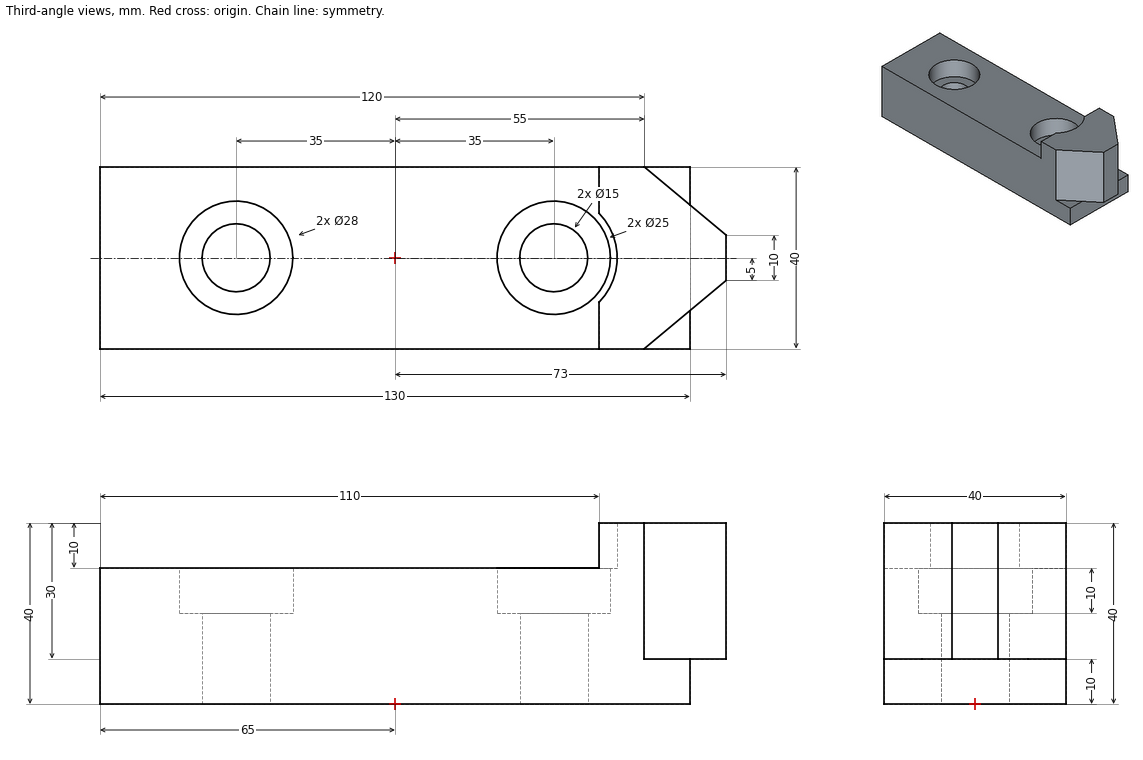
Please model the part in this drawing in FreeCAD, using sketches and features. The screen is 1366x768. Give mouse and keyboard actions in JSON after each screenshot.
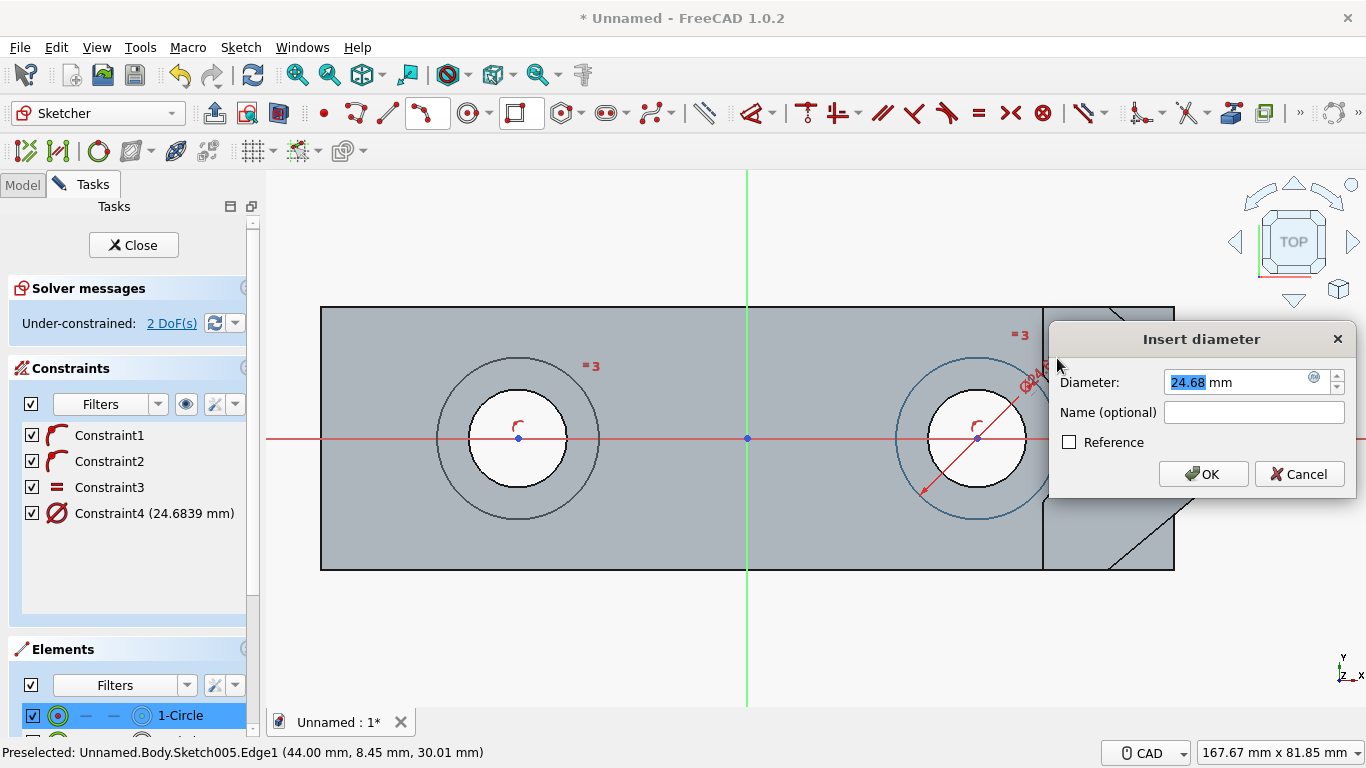
{"action": "type", "text": "25"}
{"action": "key", "text": "Return"}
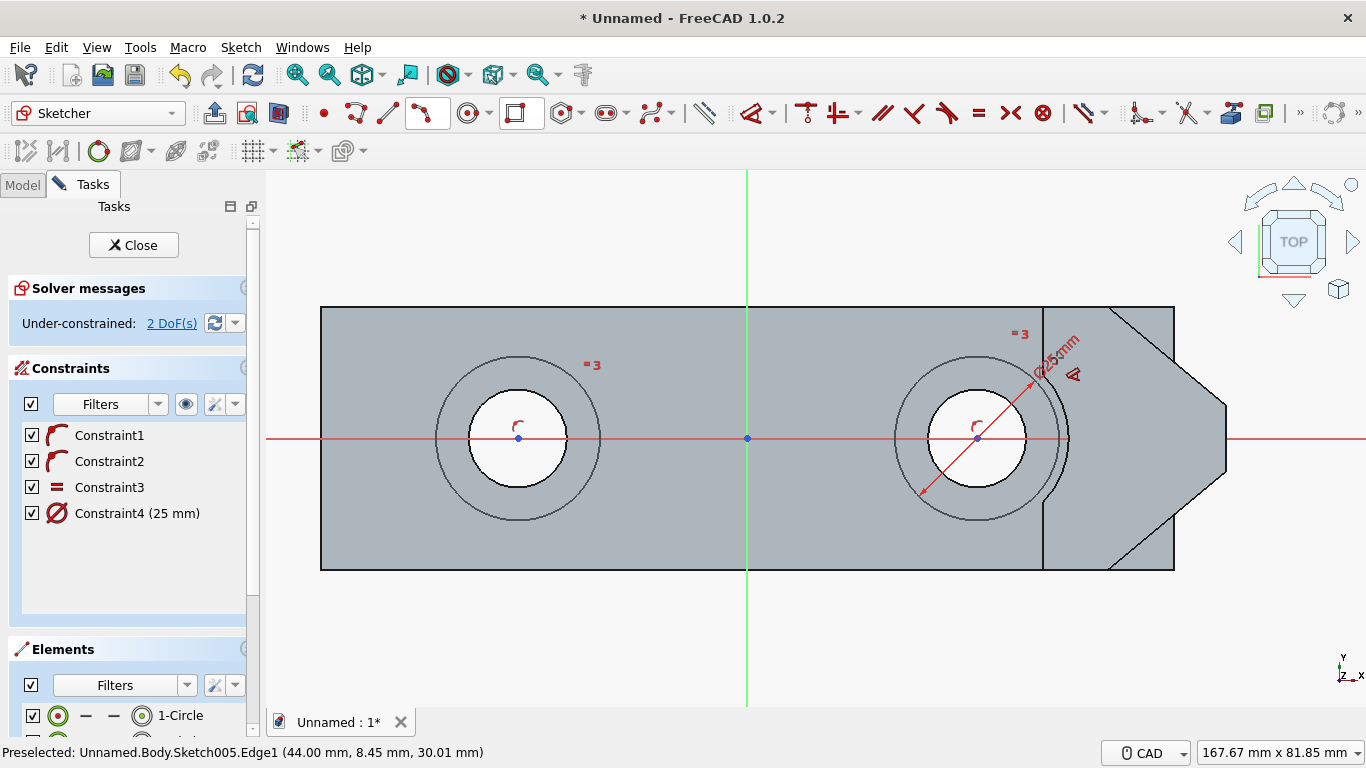
{"action": "left_click", "coordinate": [977, 438]}
{"action": "left_click", "coordinate": [862, 472]}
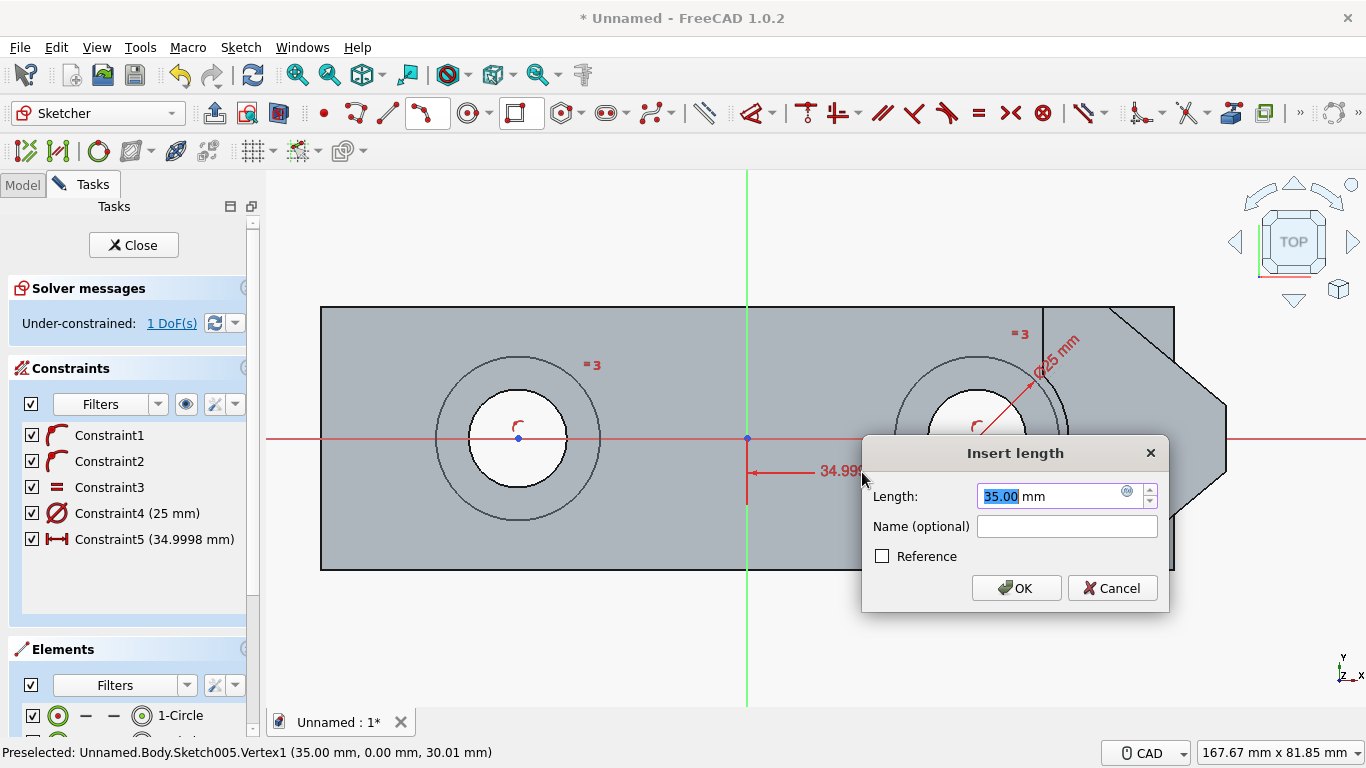
{"action": "type", "text": "35"}
{"action": "key", "text": "Return"}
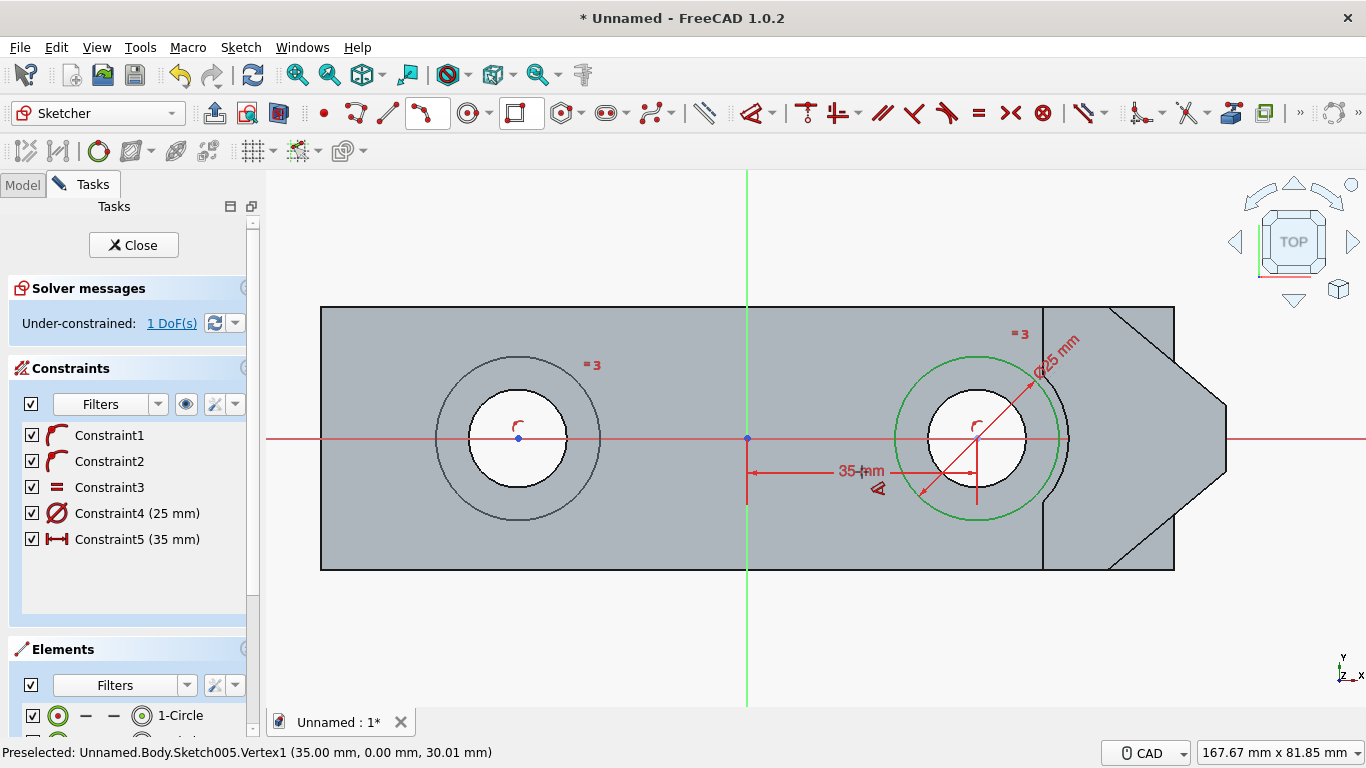
{"action": "left_click", "coordinate": [518, 438]}
{"action": "left_click", "coordinate": [633, 472]}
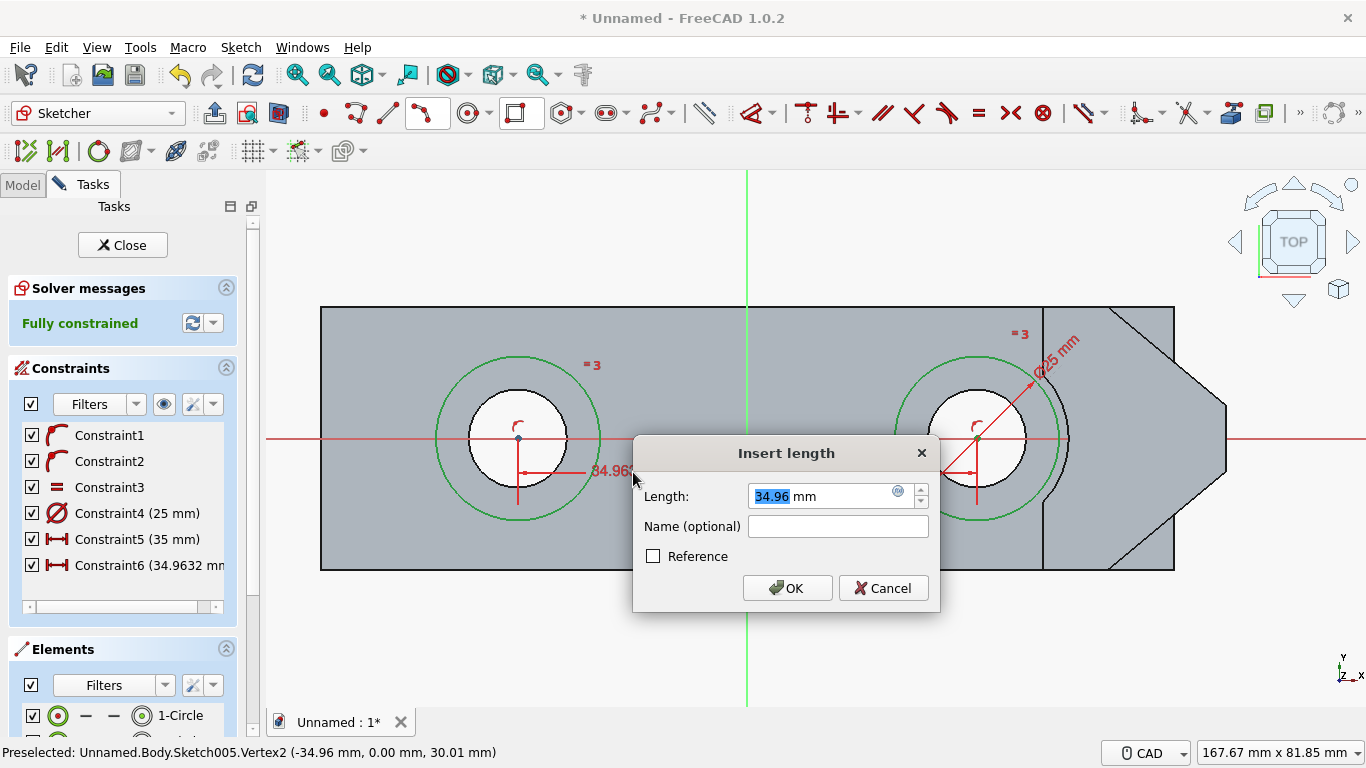
{"action": "type", "text": "35"}
{"action": "key", "text": "Return"}
{"action": "key", "text": "Escape"}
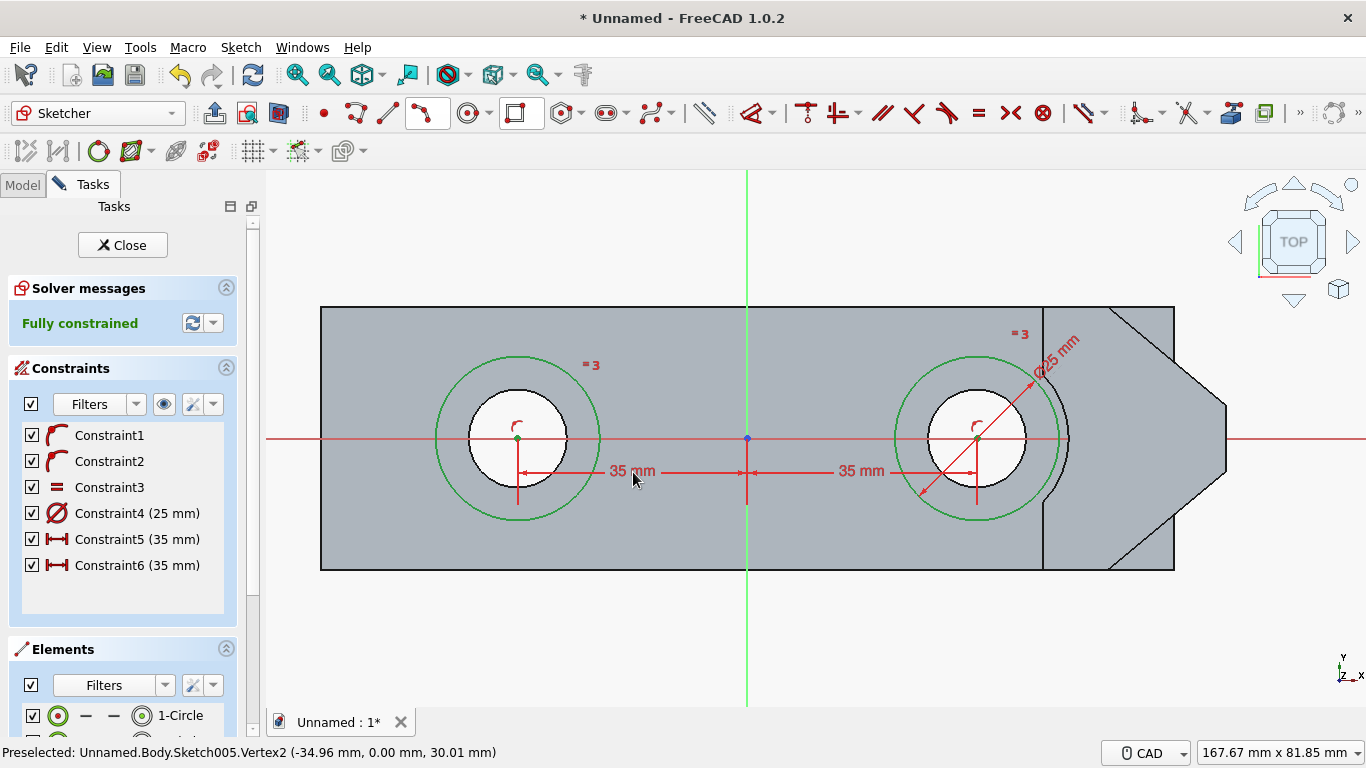
{"action": "left_click", "coordinate": [123, 245]}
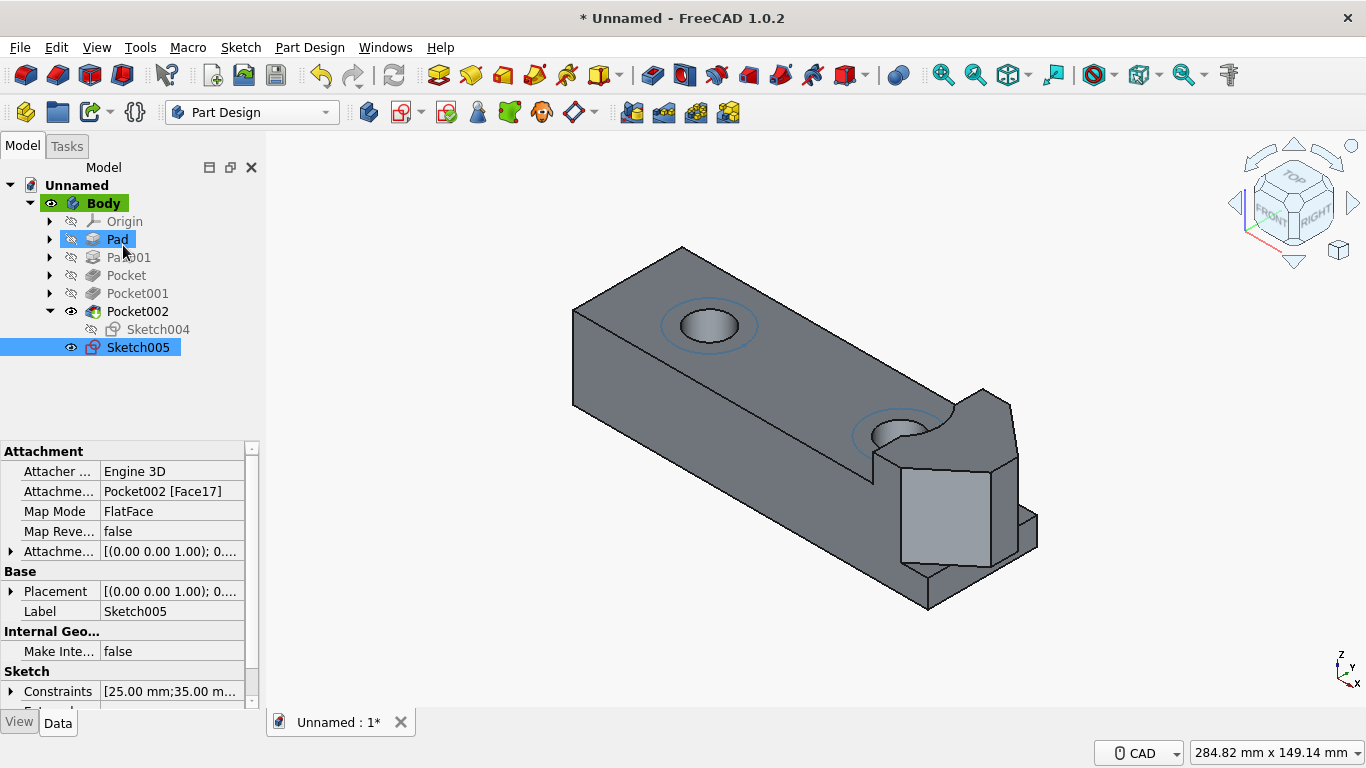
{"action": "left_click", "coordinate": [654, 76]}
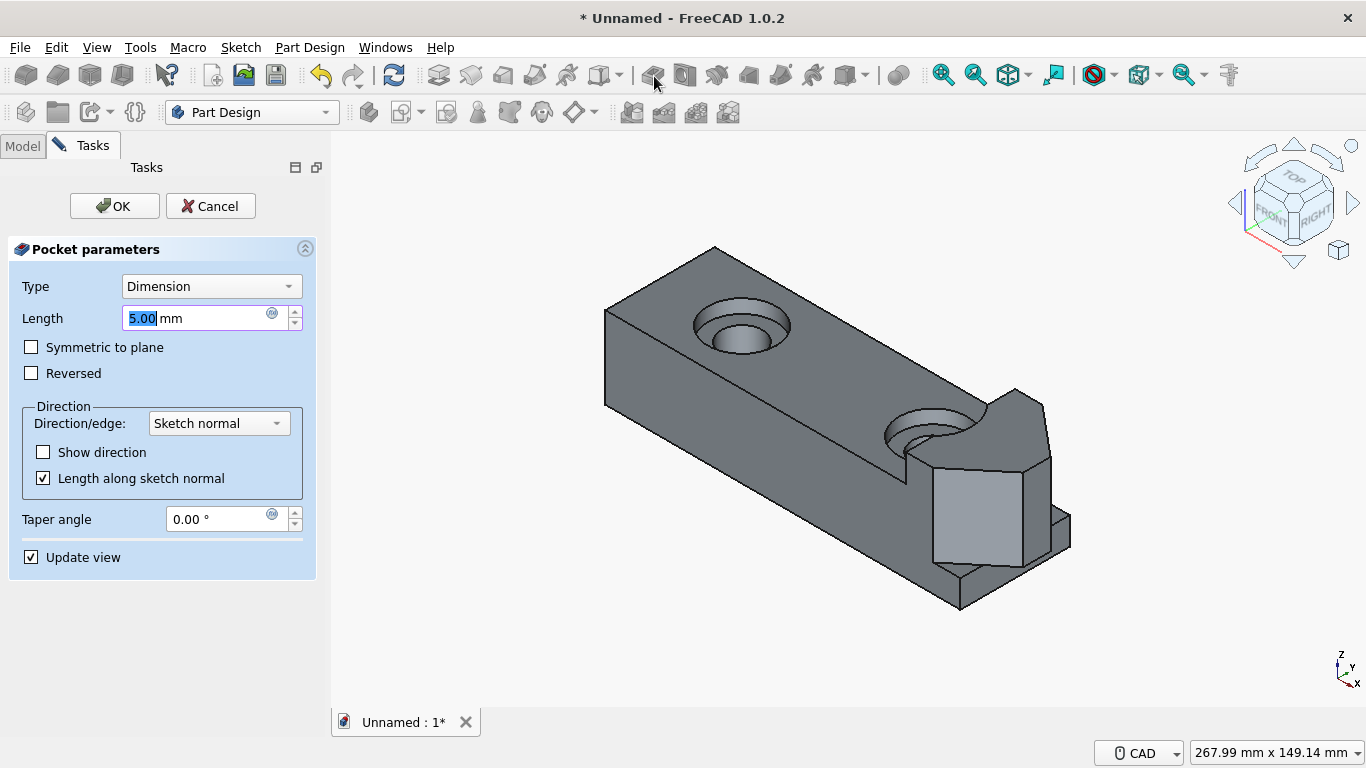
{"action": "type", "text": "10"}
{"action": "key", "text": "Tab"}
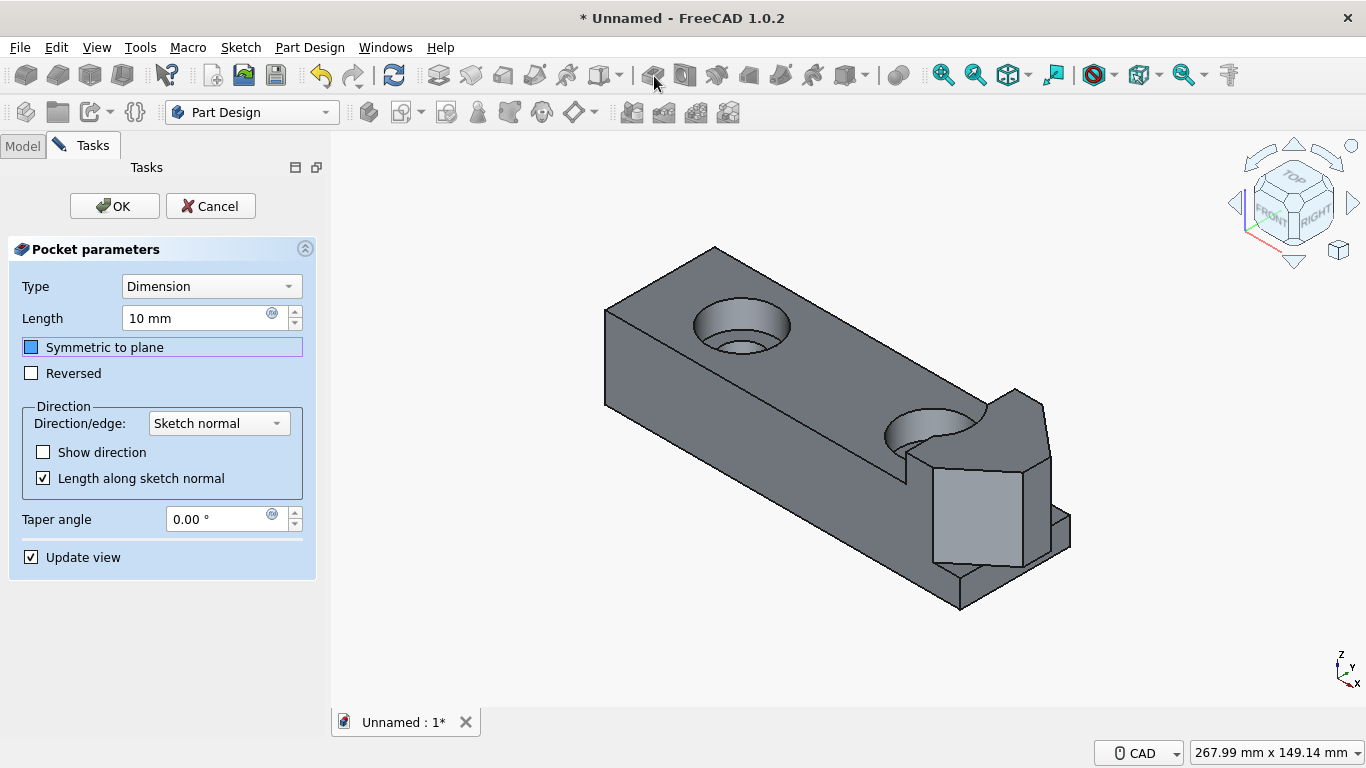
{"action": "left_click", "coordinate": [115, 206]}